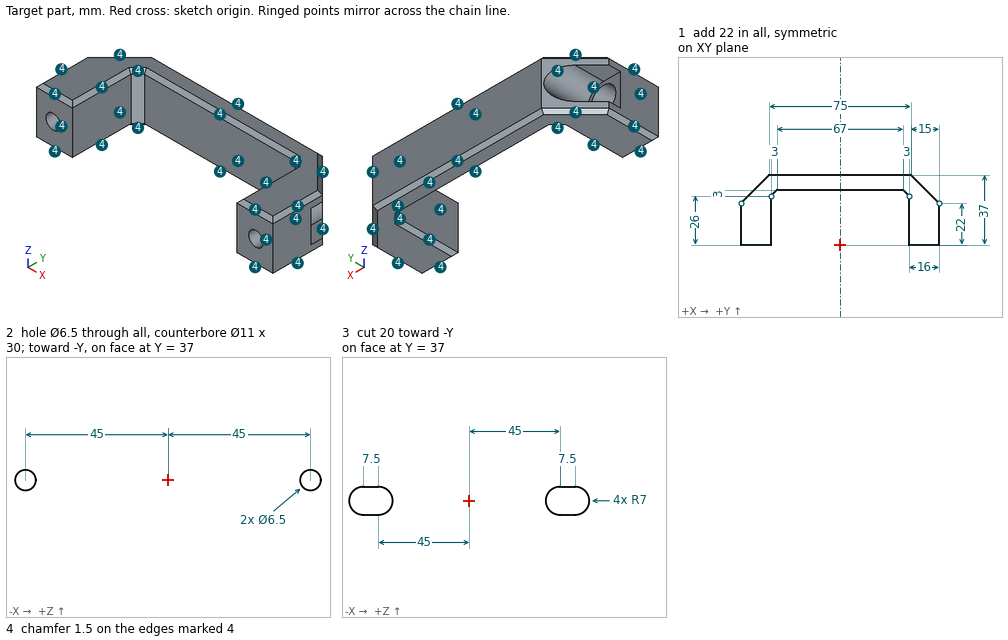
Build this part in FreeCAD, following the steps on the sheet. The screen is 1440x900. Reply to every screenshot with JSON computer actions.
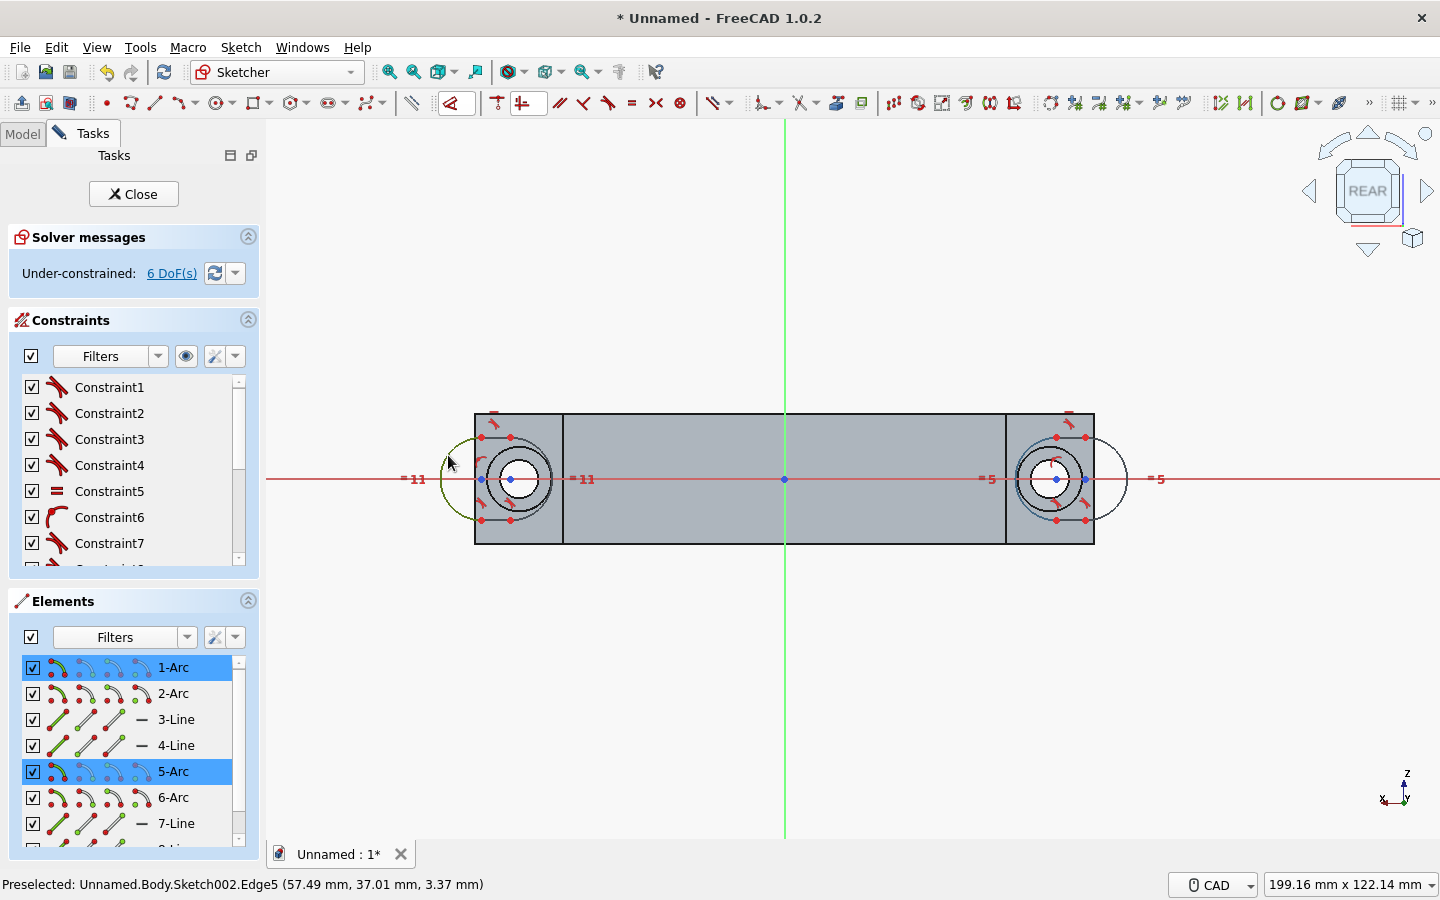
{"action": "left_click", "coordinate": [632, 104]}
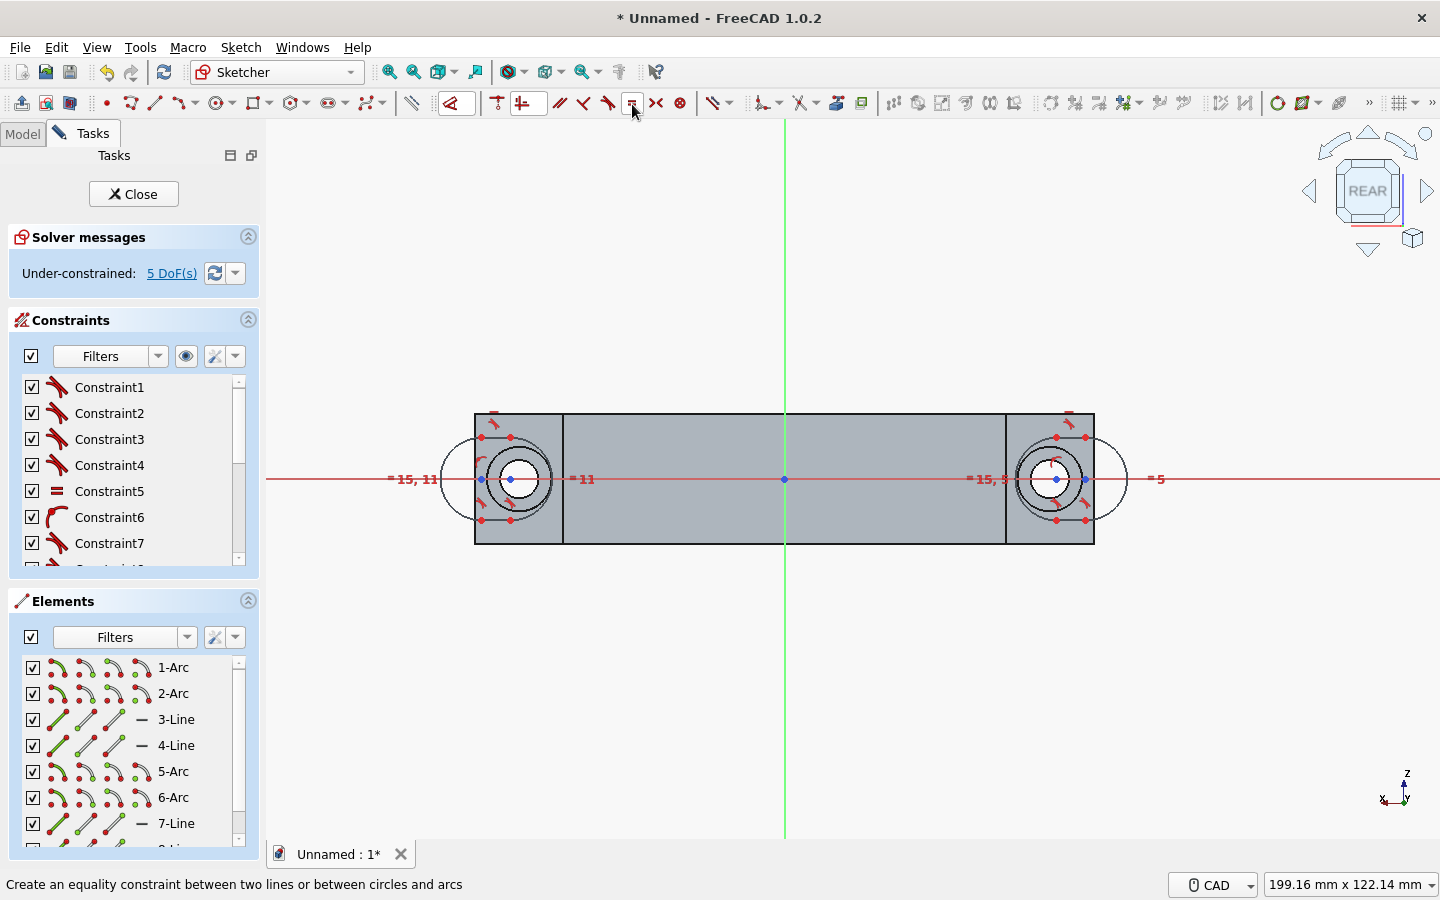
{"action": "left_click", "coordinate": [1023, 455]}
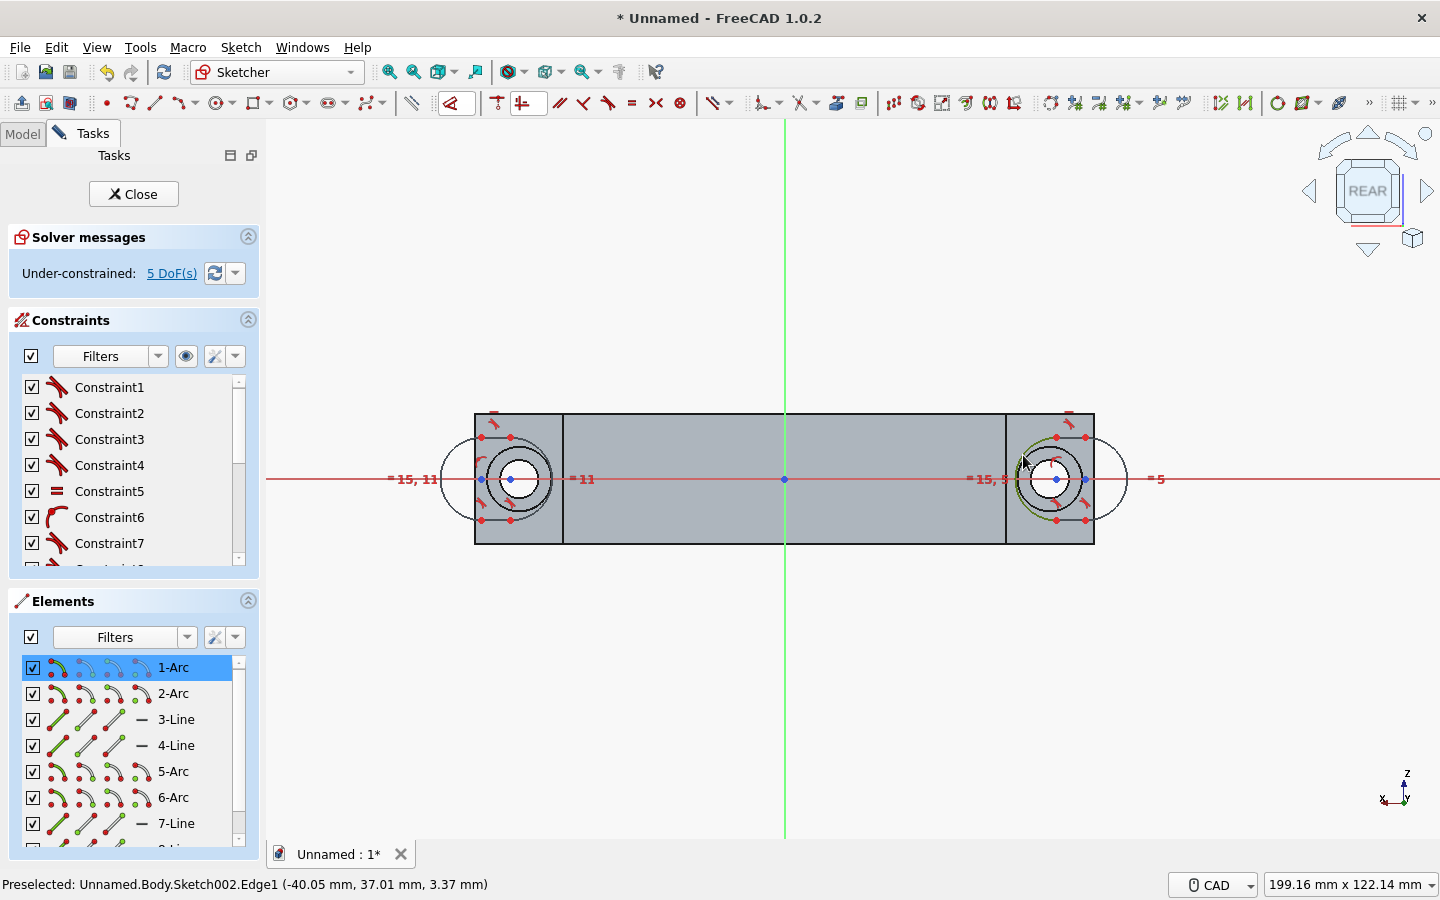
{"action": "left_click", "coordinate": [470, 104]}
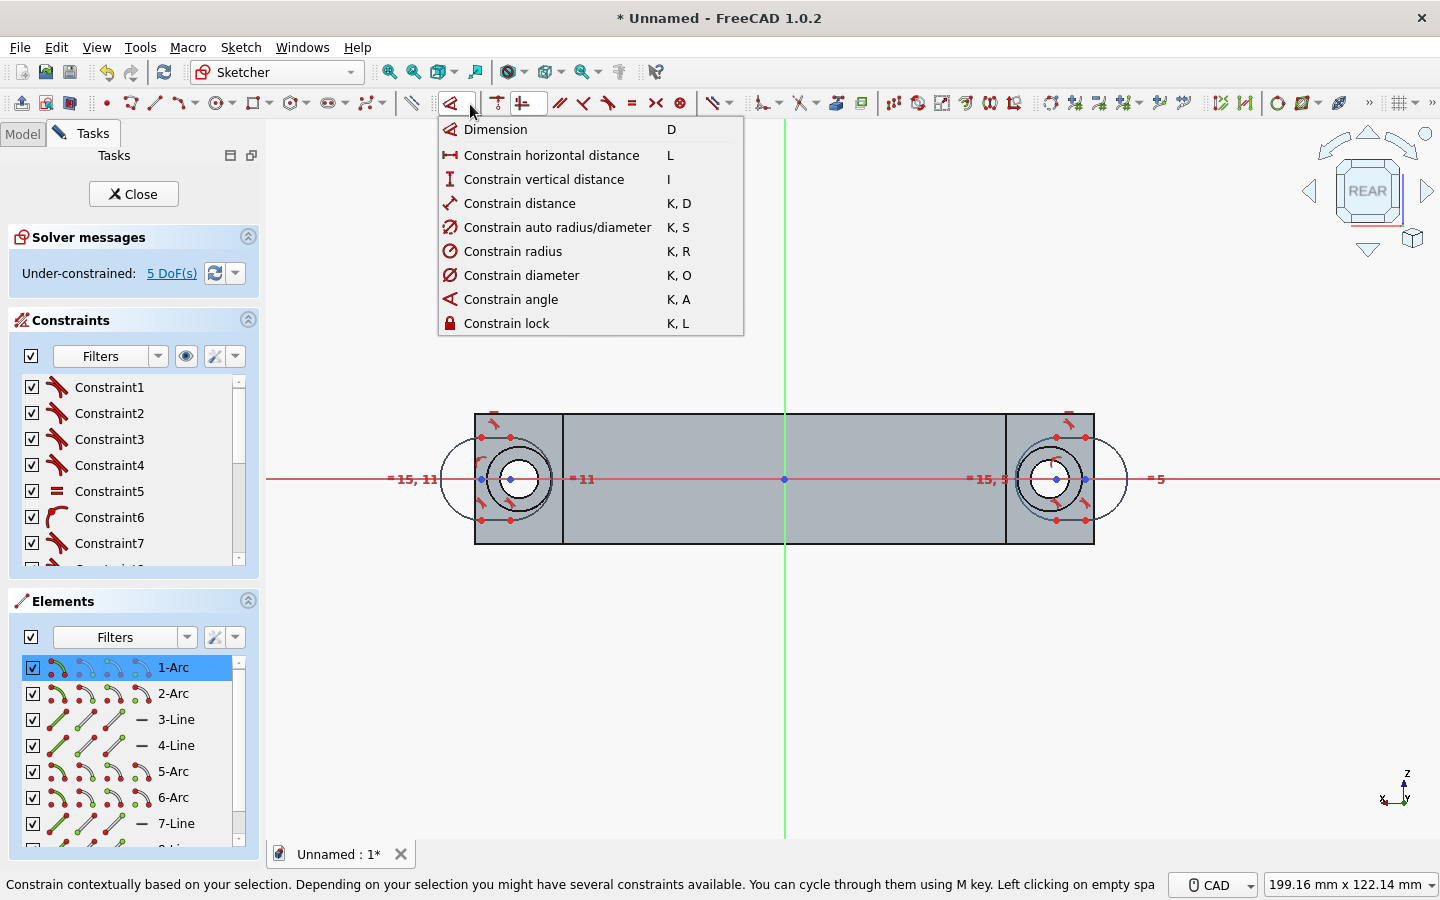
{"action": "left_click", "coordinate": [591, 251]}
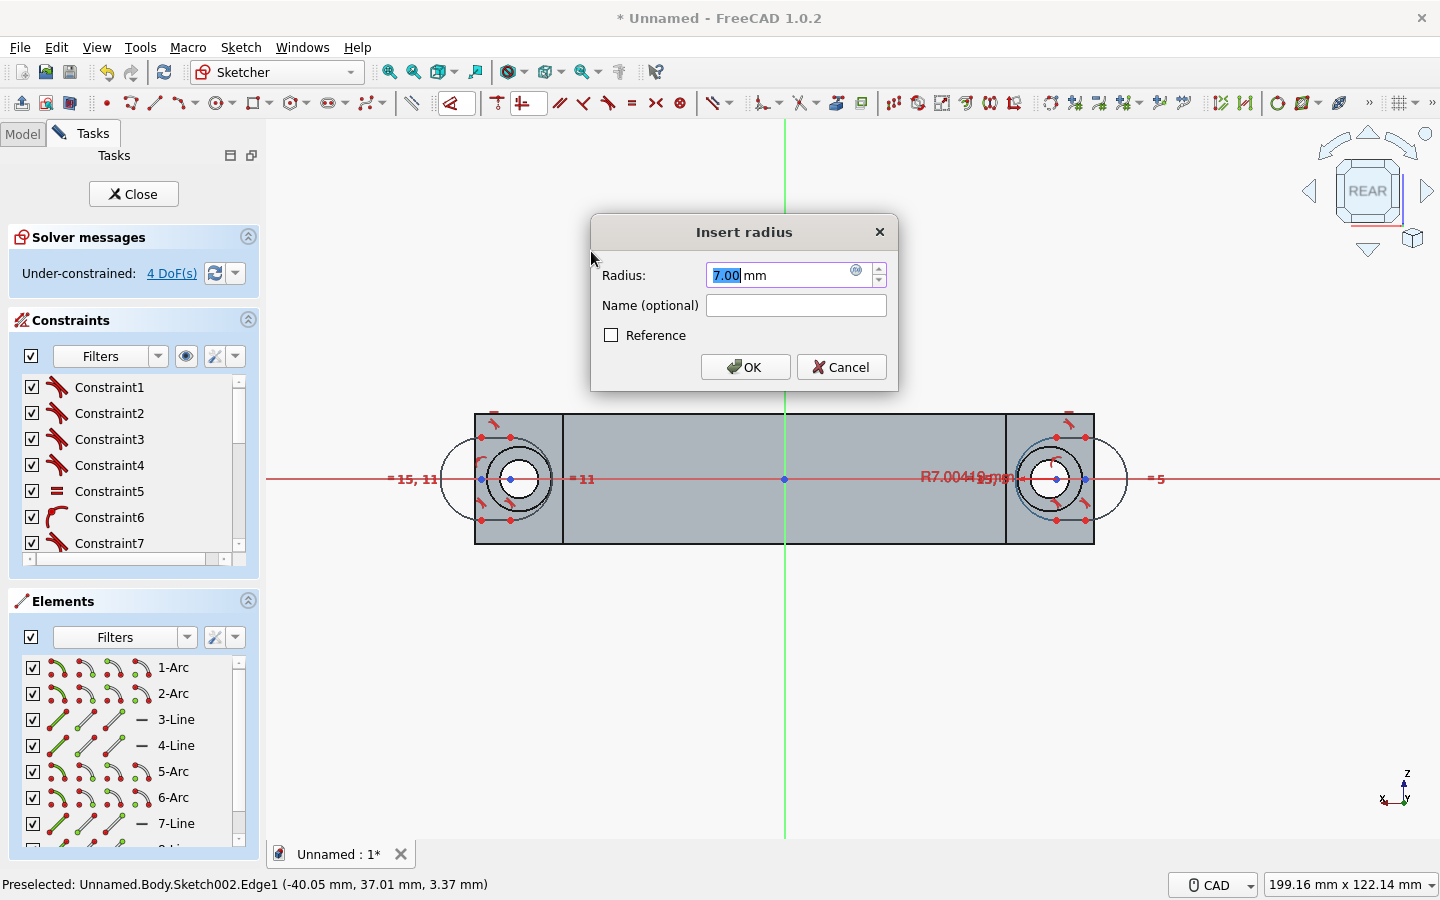
{"action": "type", "text": "7"}
{"action": "key", "text": "Return"}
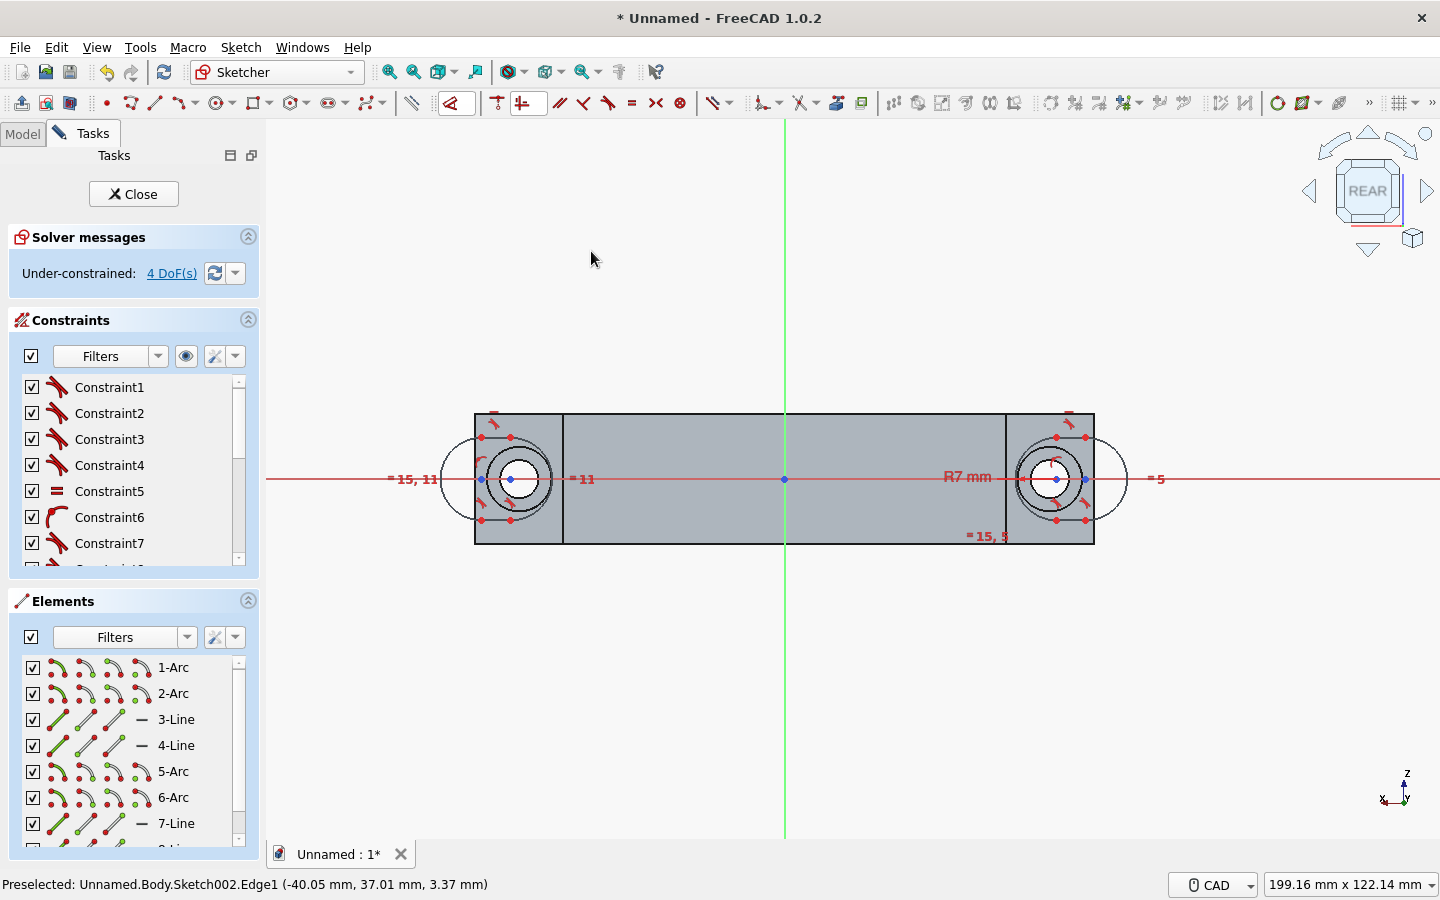
{"action": "left_click", "coordinate": [1068, 438]}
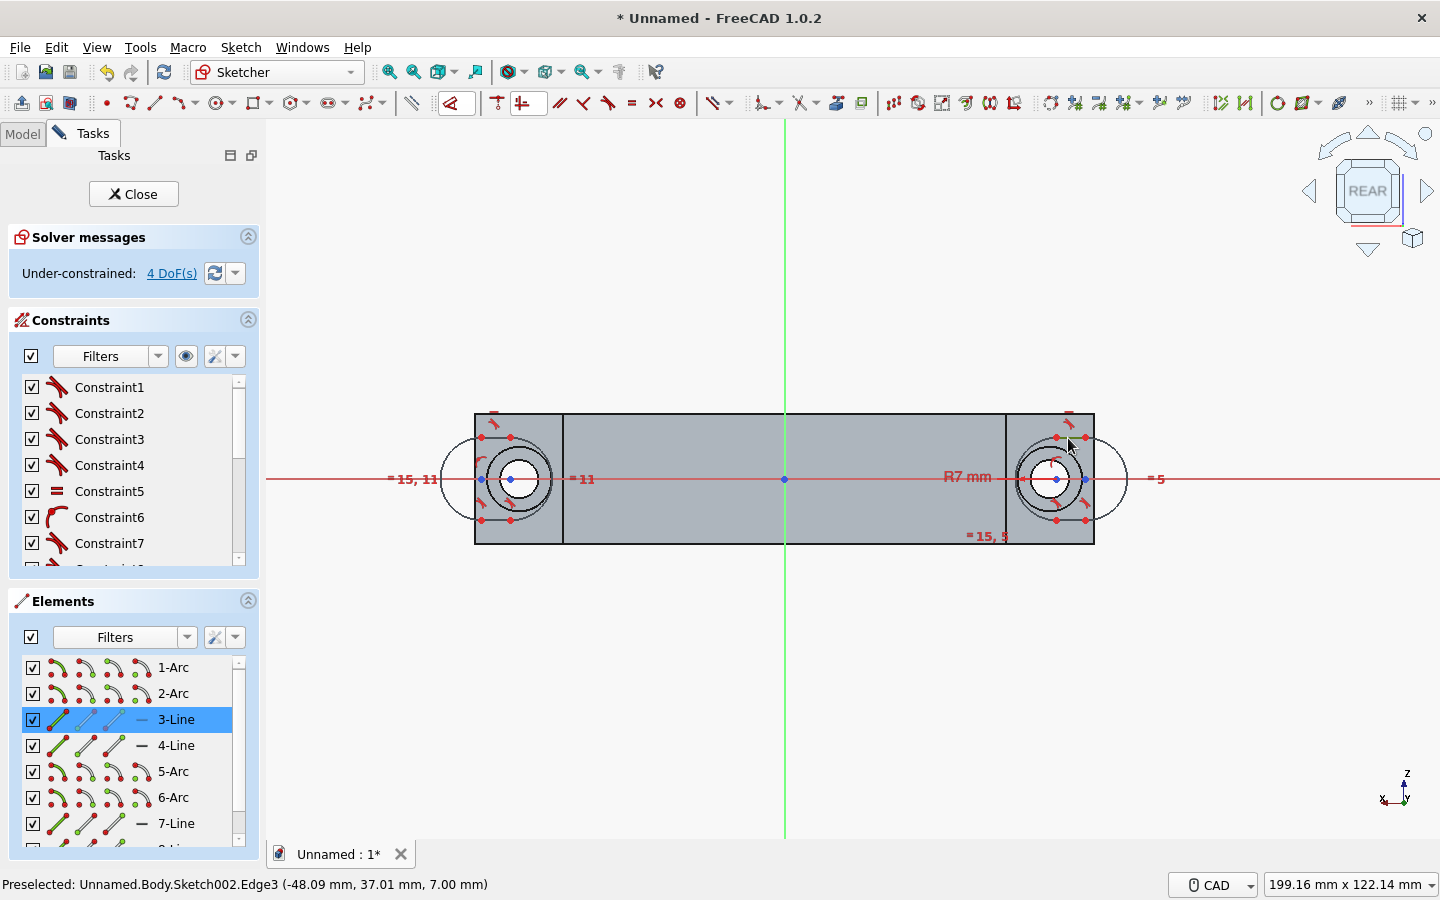
{"action": "key", "text": "l"}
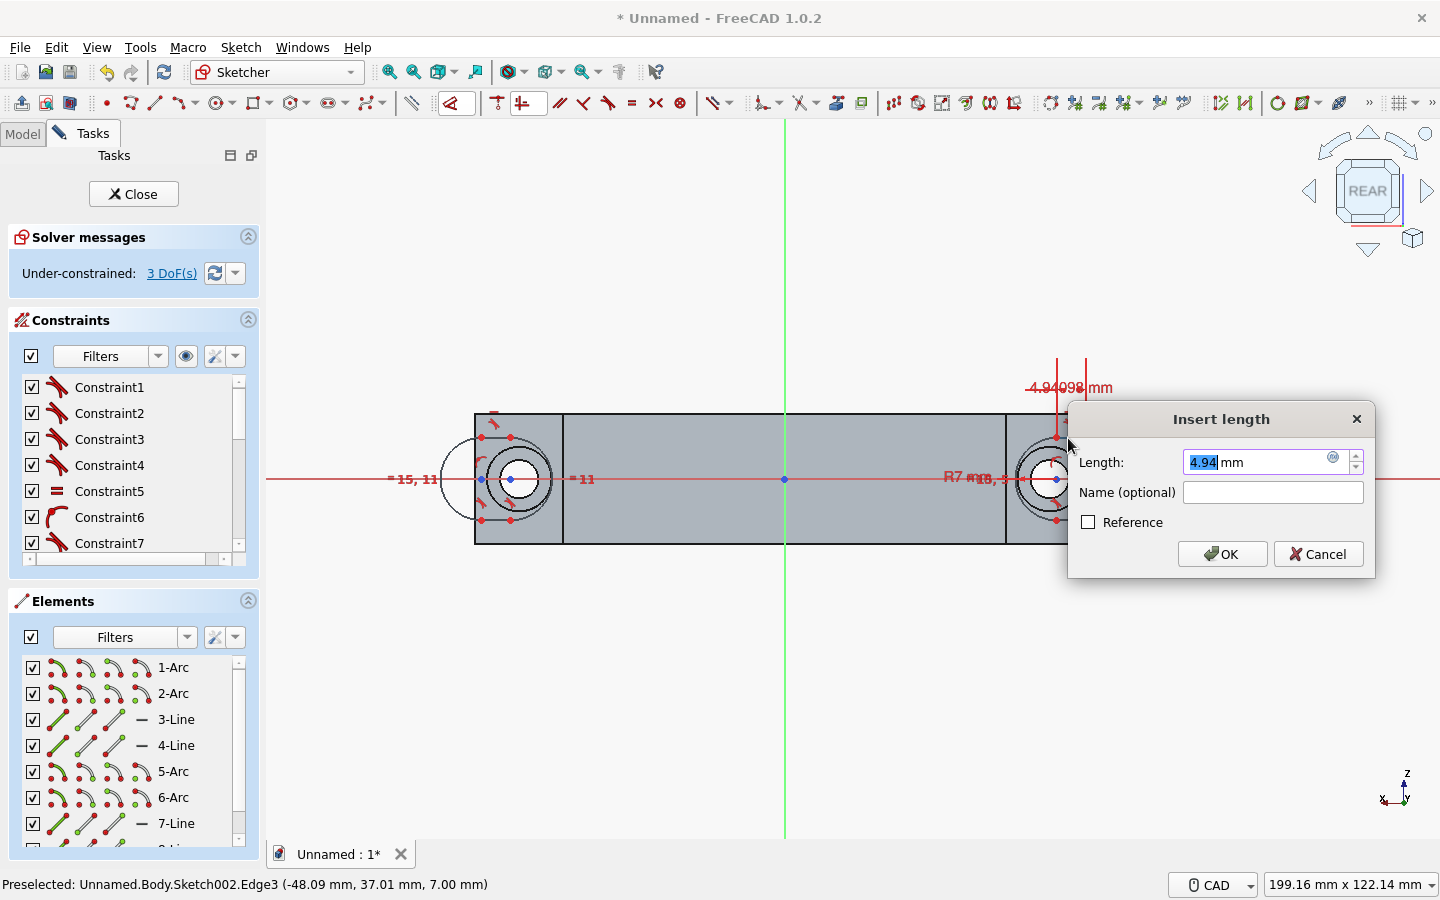
{"action": "type", "text": "7.5"}
{"action": "key", "text": "Return"}